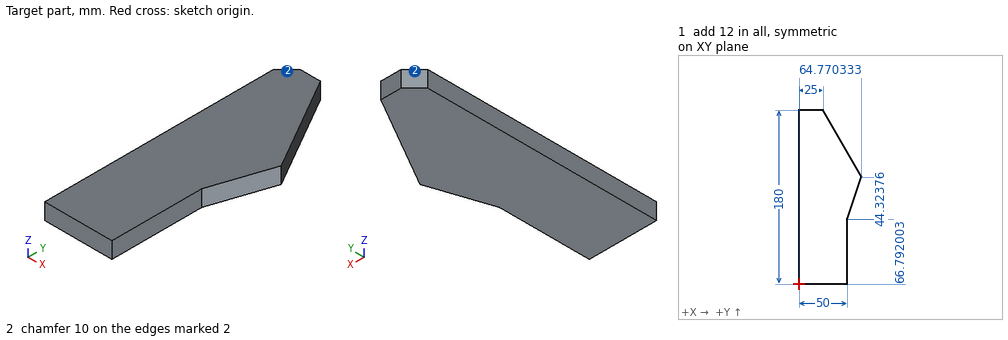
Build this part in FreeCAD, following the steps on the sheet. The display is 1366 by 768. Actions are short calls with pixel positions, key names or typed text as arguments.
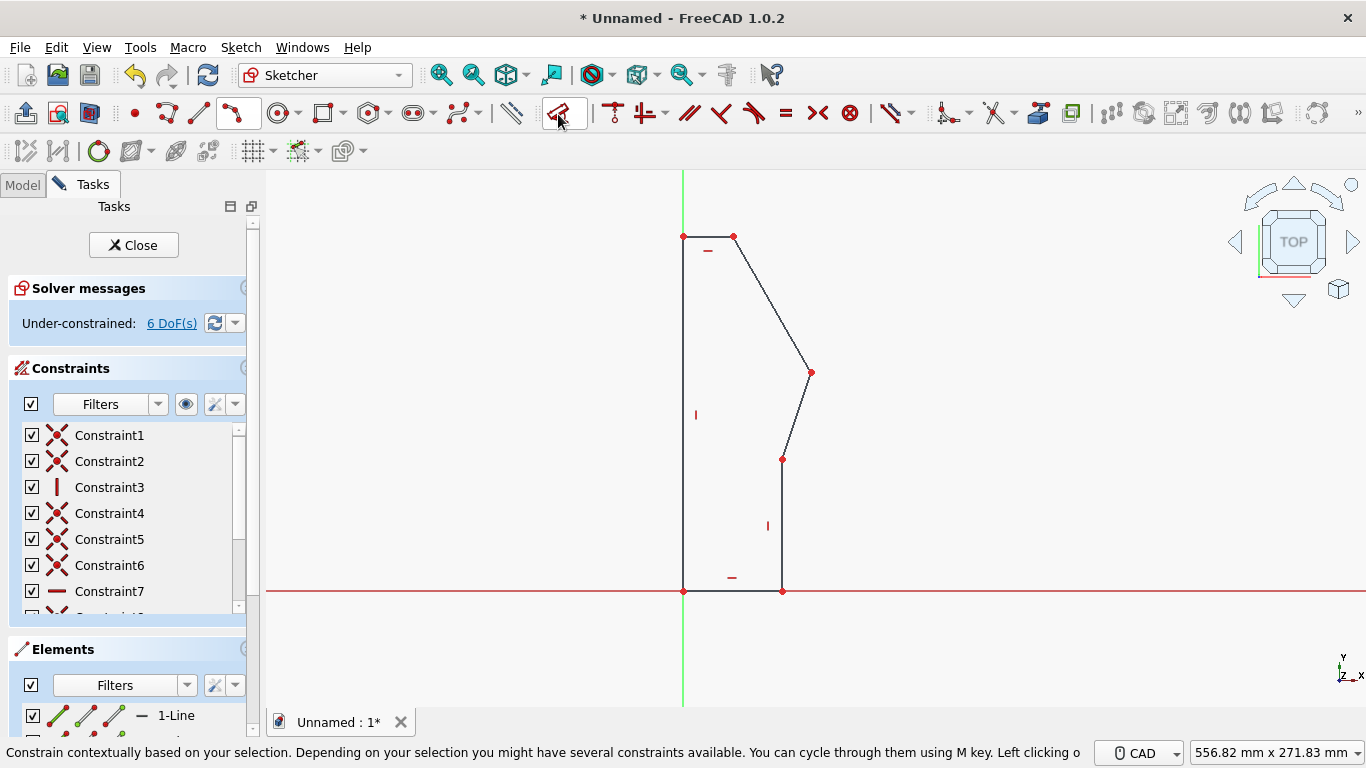
click(713, 591)
click(733, 625)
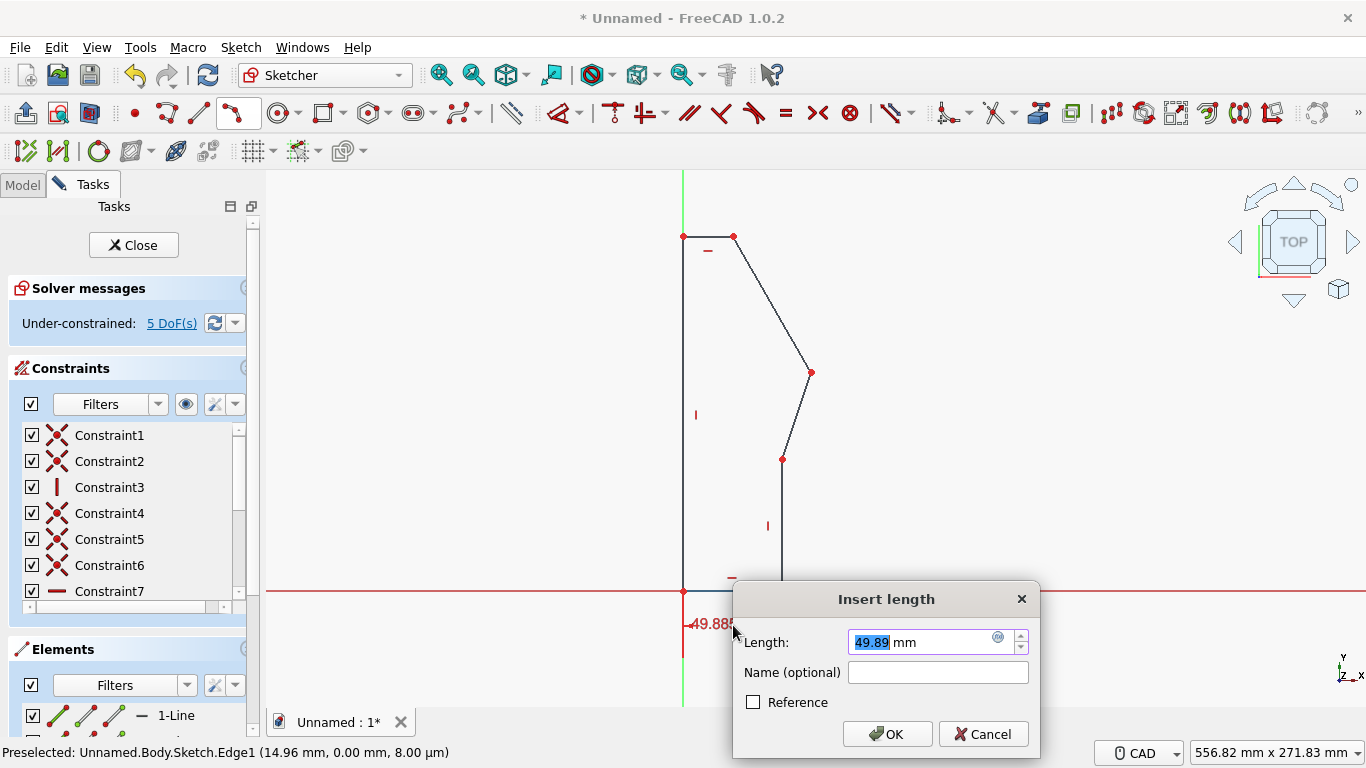
text(50)
key(Return)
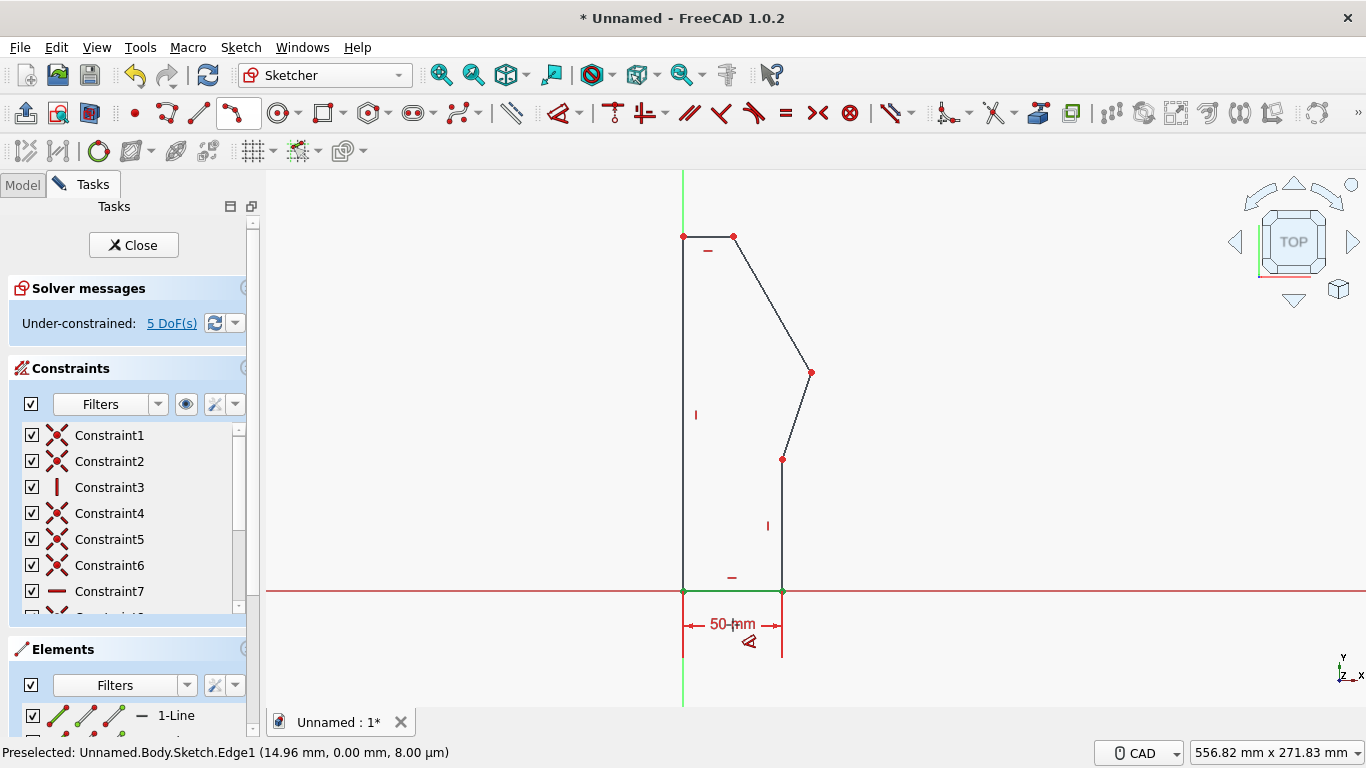
click(718, 237)
click(708, 203)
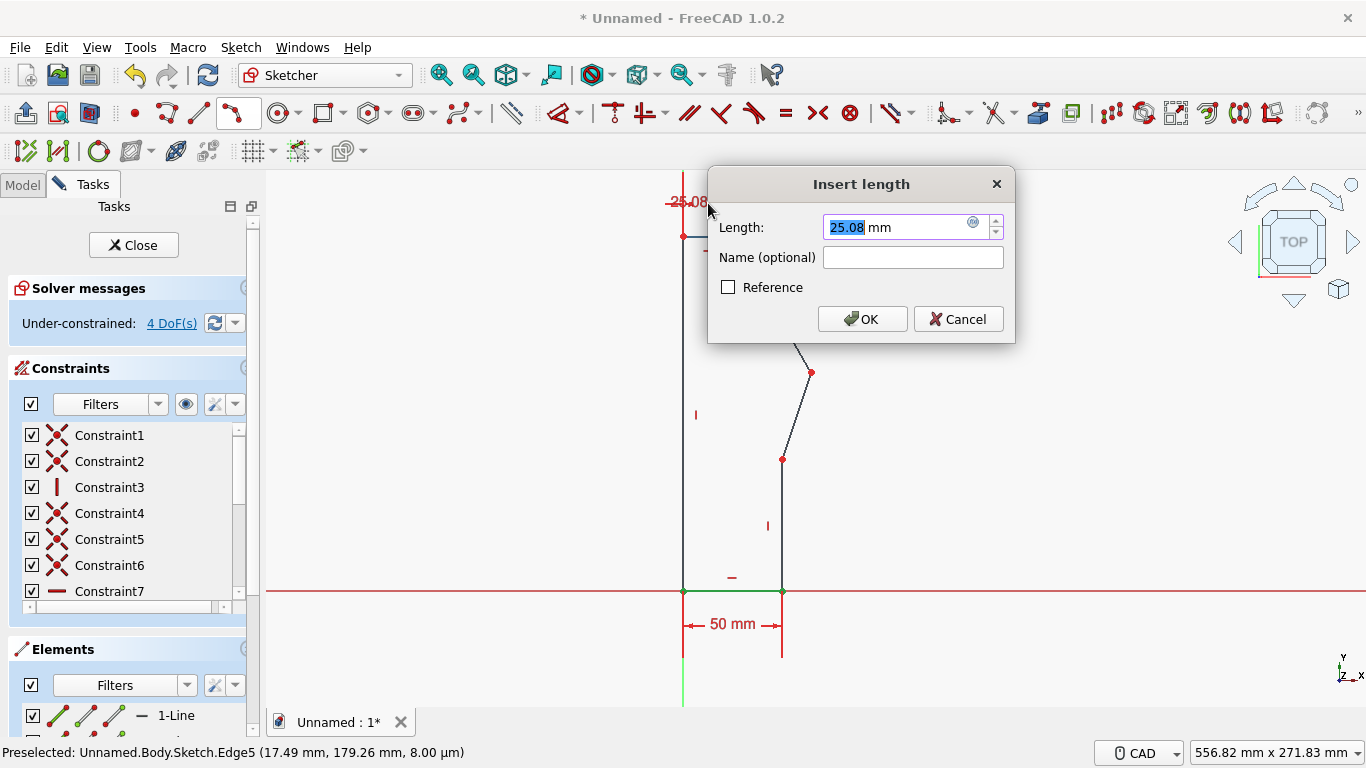
text(25)
key(Return)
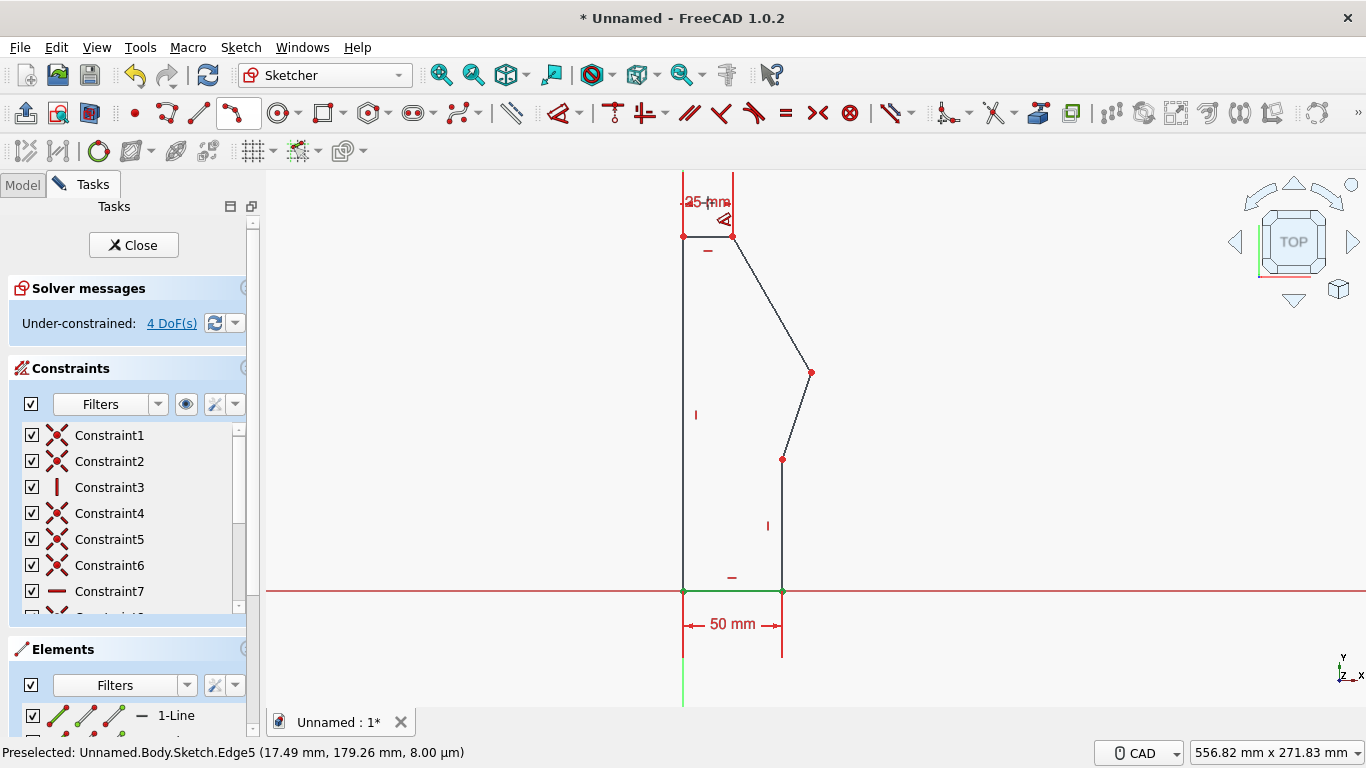
click(683, 343)
click(649, 414)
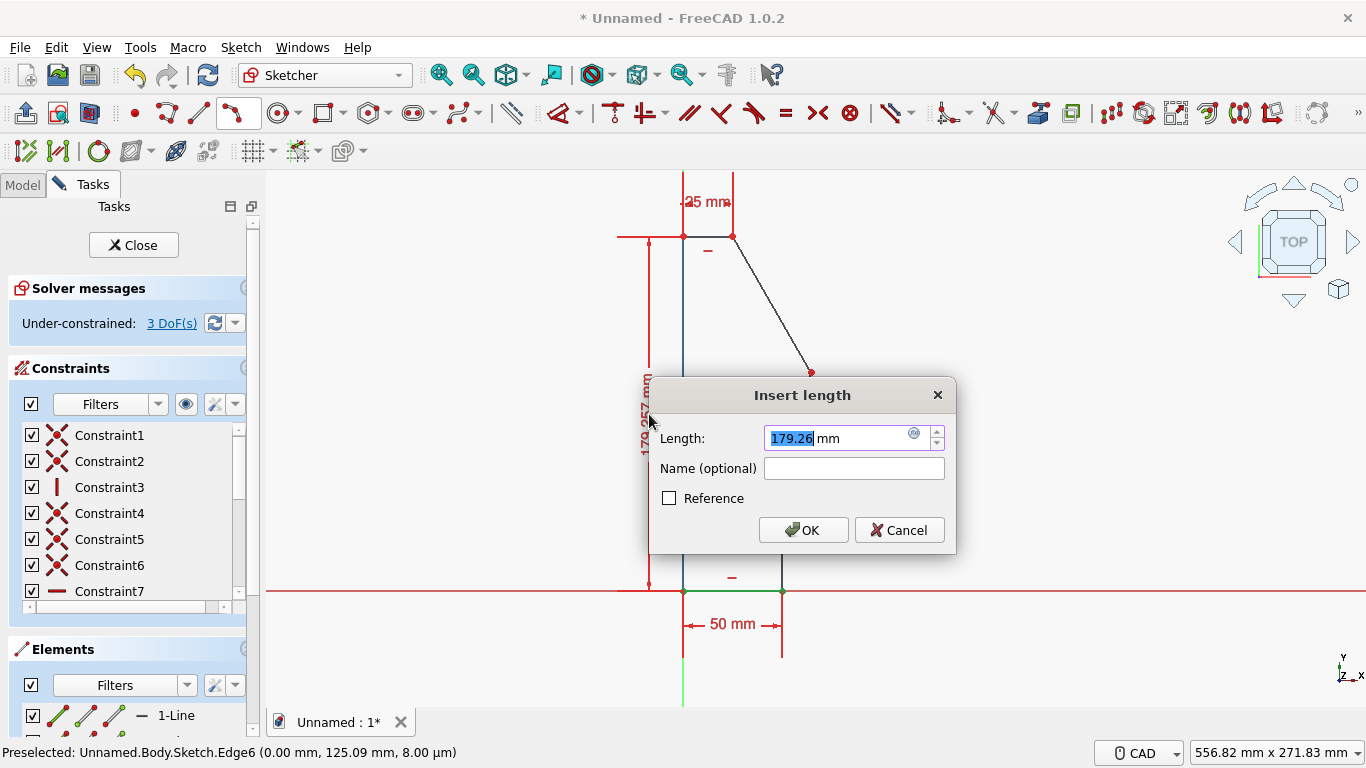
text(180)
key(Return)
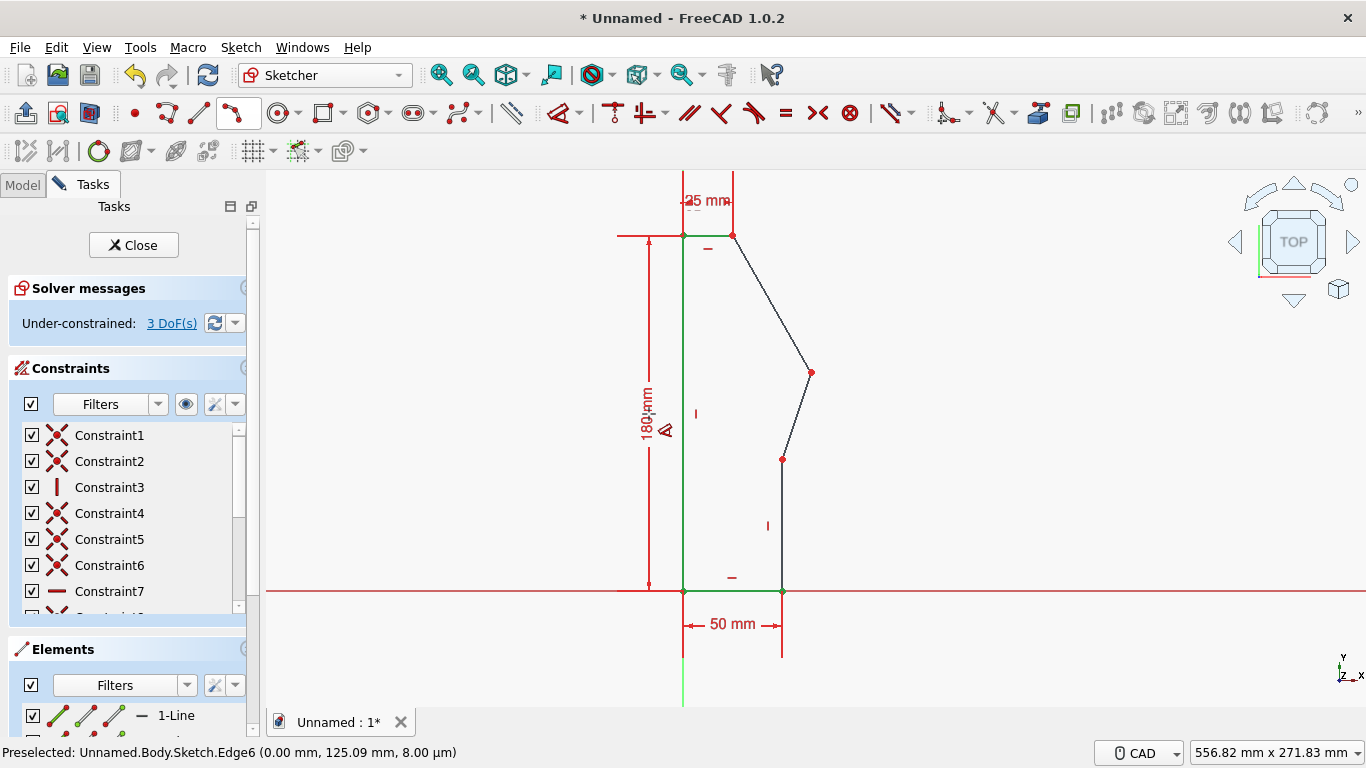
click(782, 552)
click(816, 526)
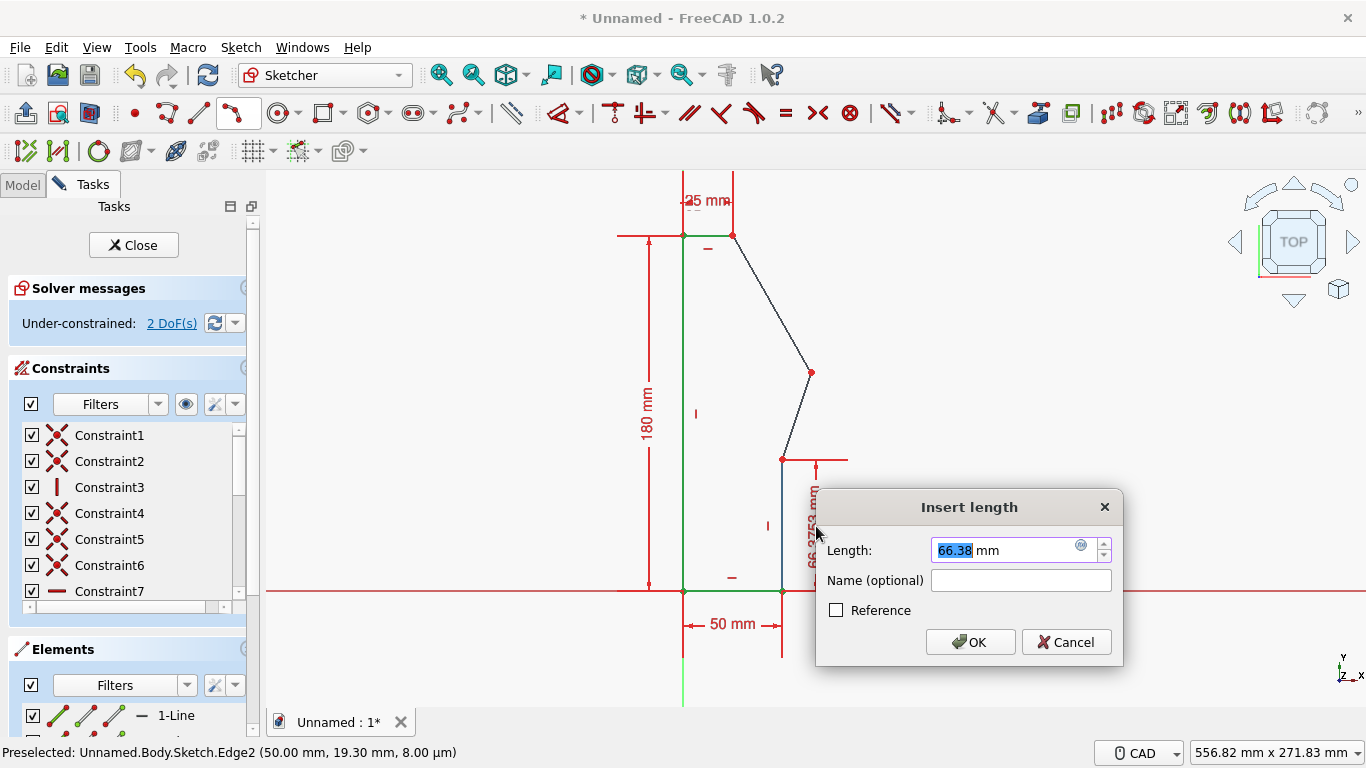
text(66.792003)
key(Return)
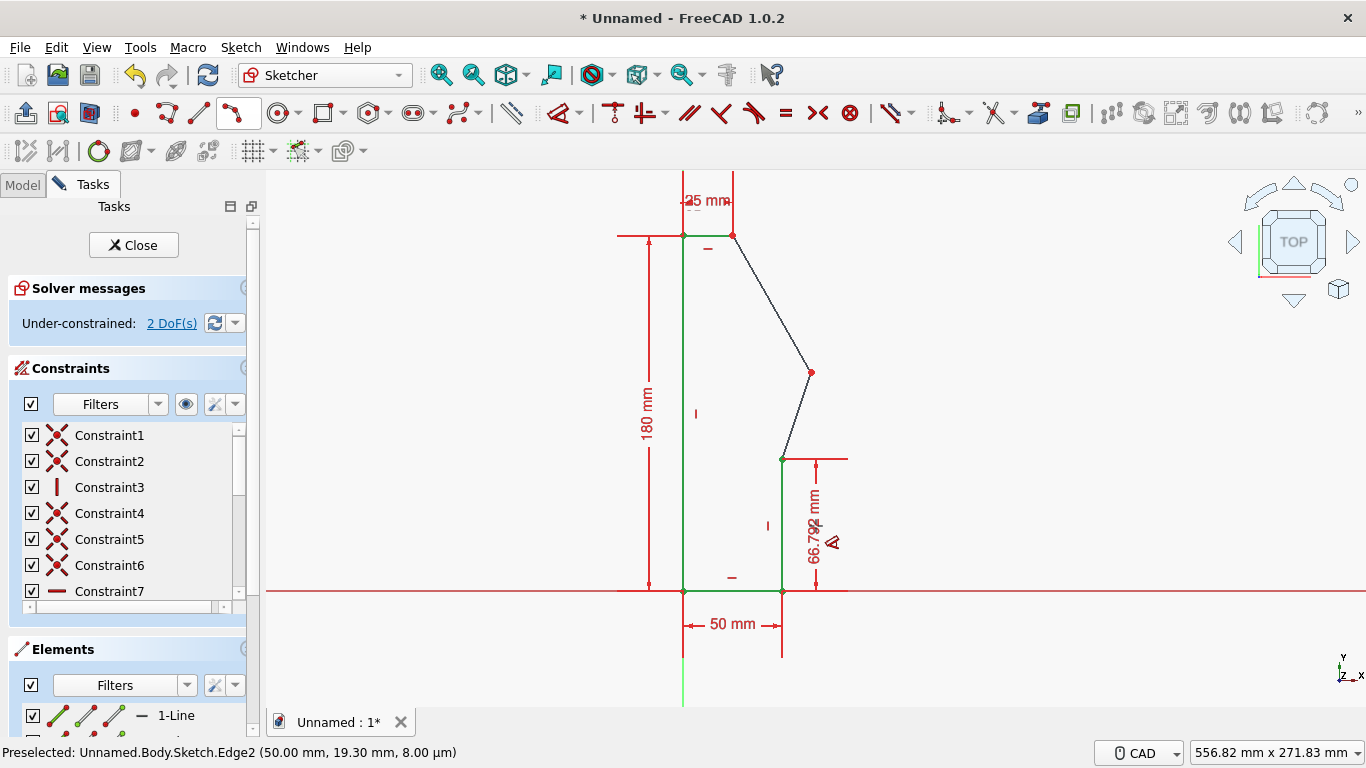
click(791, 433)
click(845, 416)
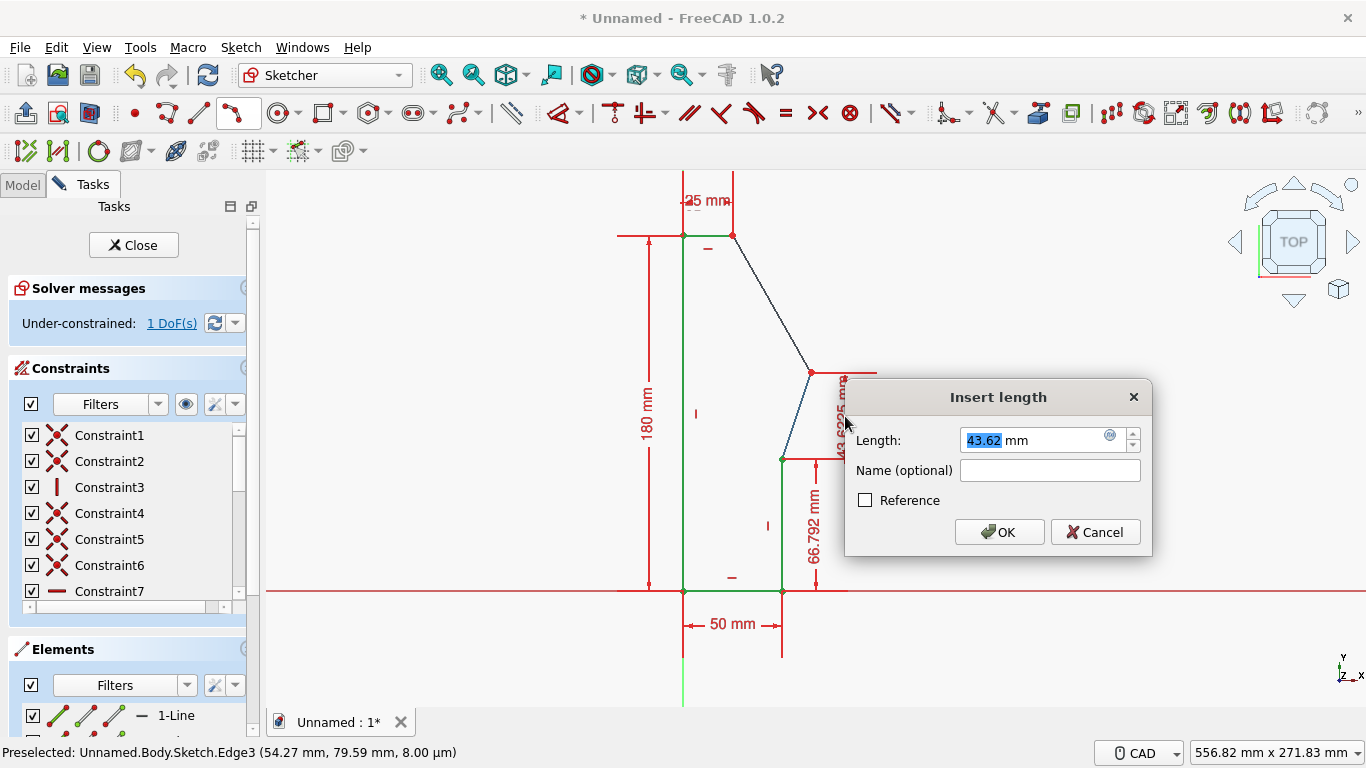
text(44.32376)
key(Return)